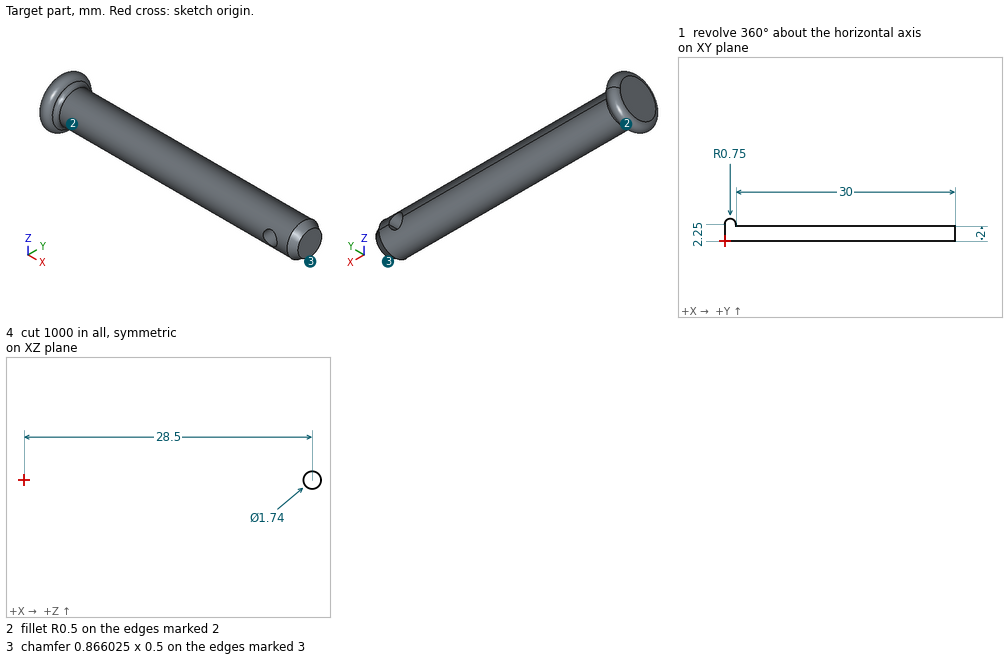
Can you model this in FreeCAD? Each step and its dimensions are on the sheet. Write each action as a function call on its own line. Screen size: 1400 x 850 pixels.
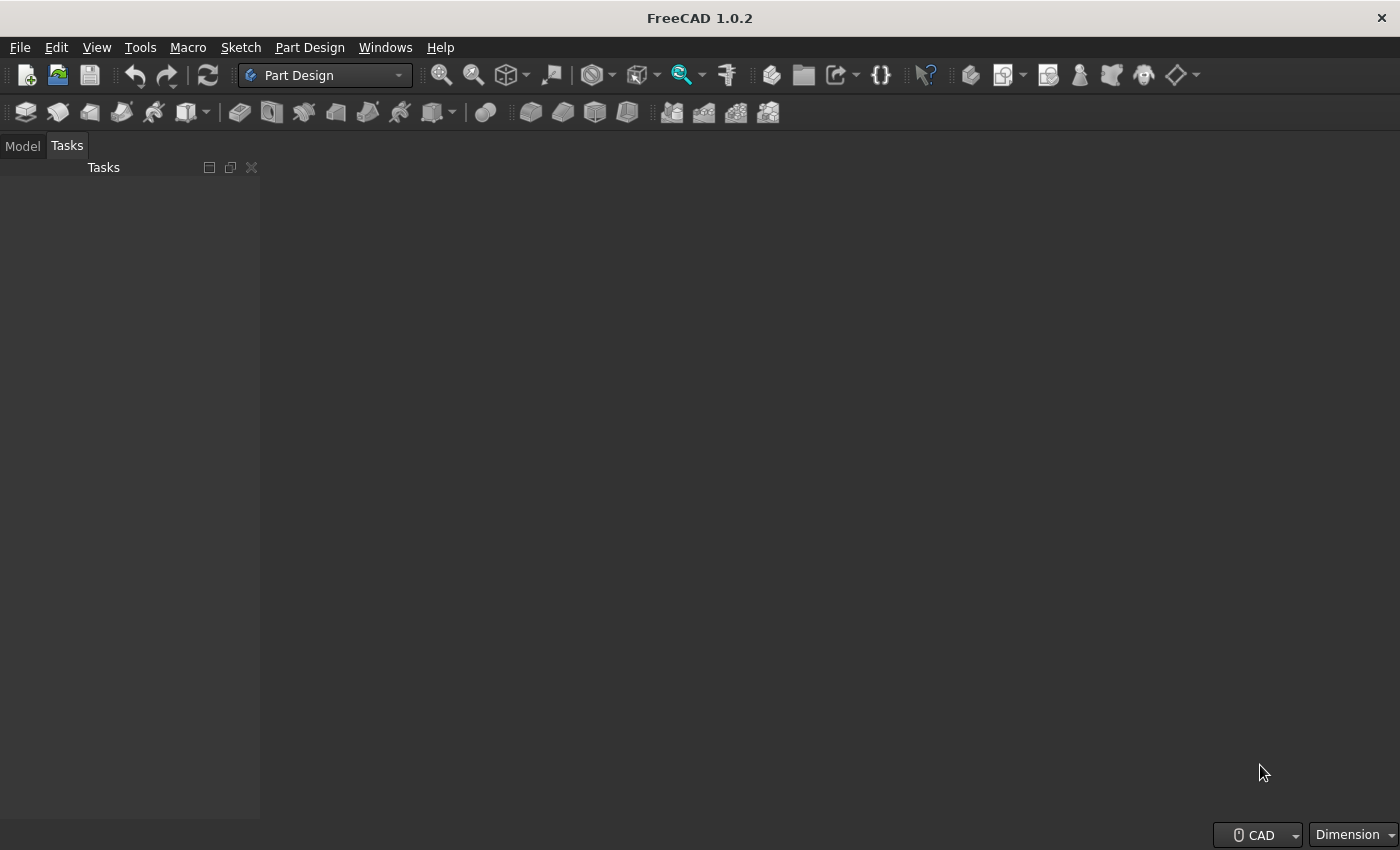
click(26, 76)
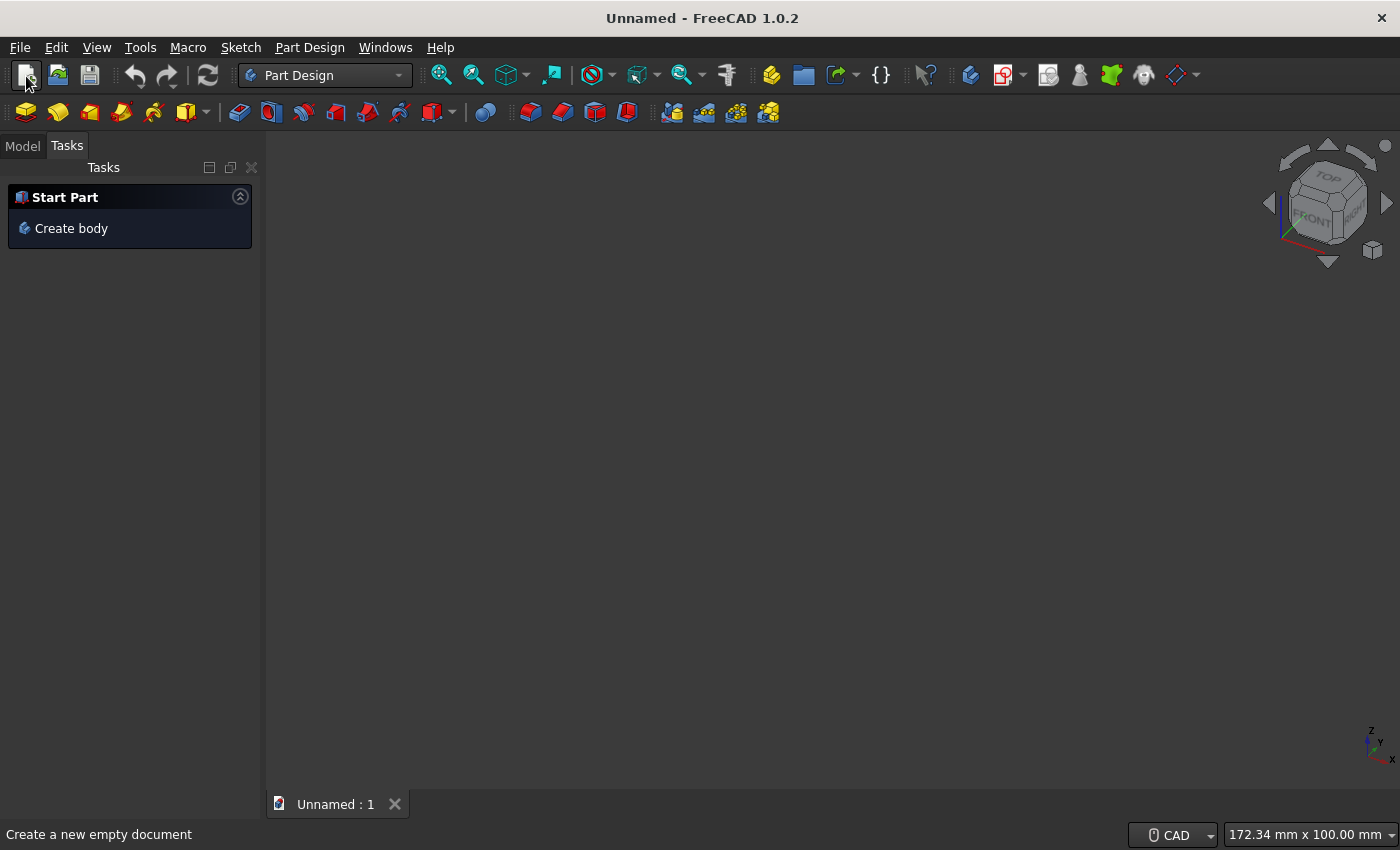
click(1004, 76)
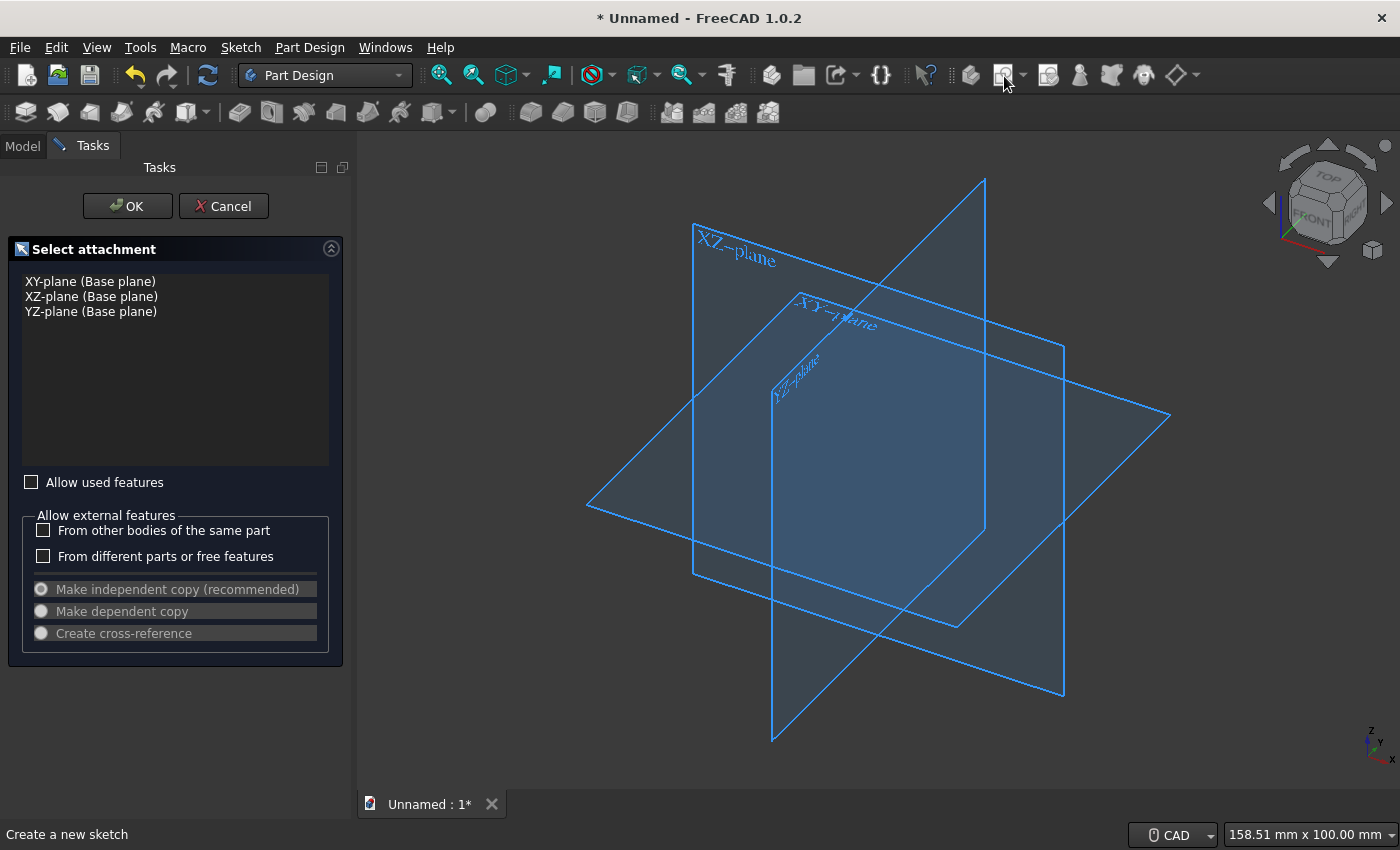
click(82, 282)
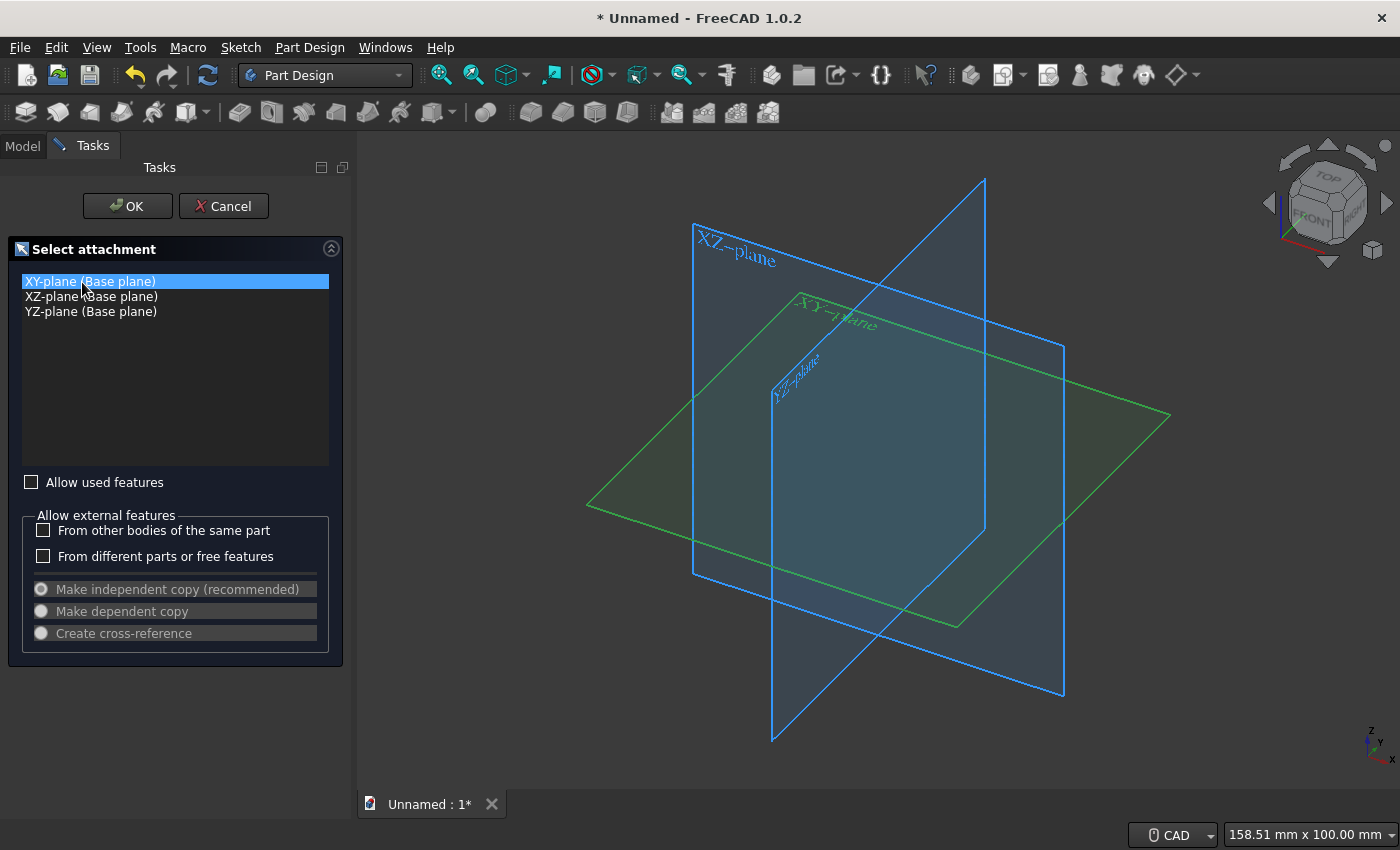
click(128, 206)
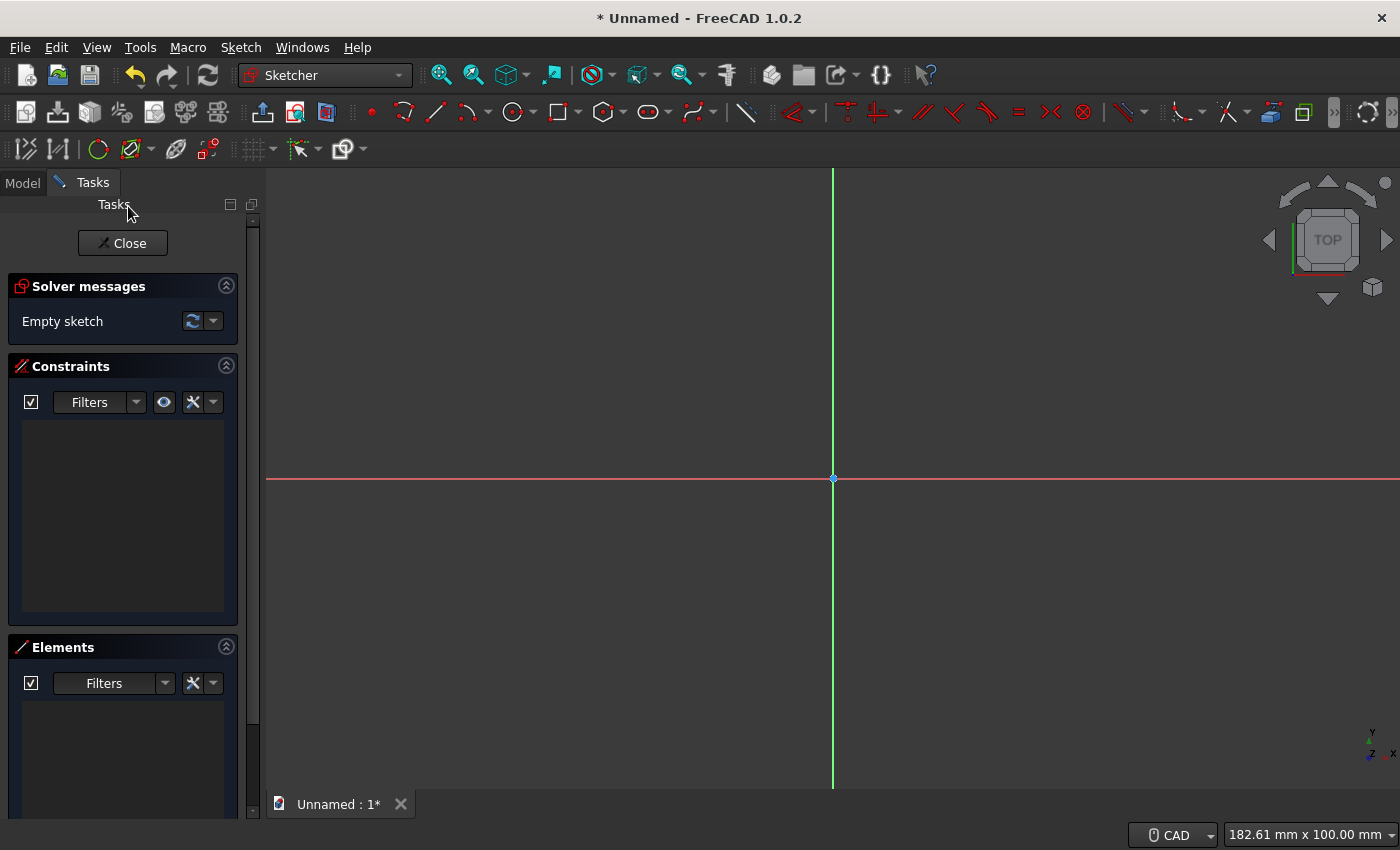
scroll(1002, 465, up, 6)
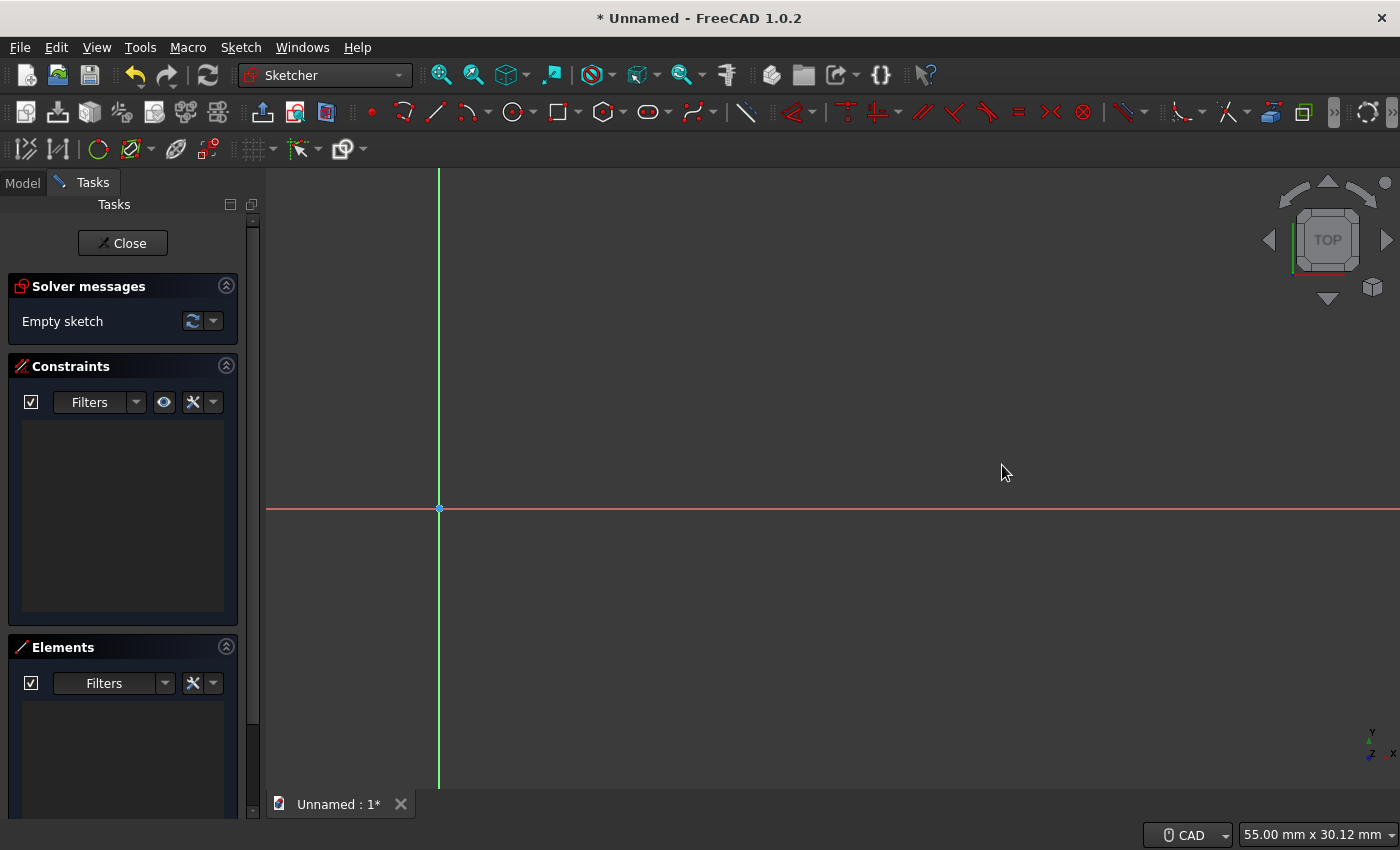
key(g)
key(m)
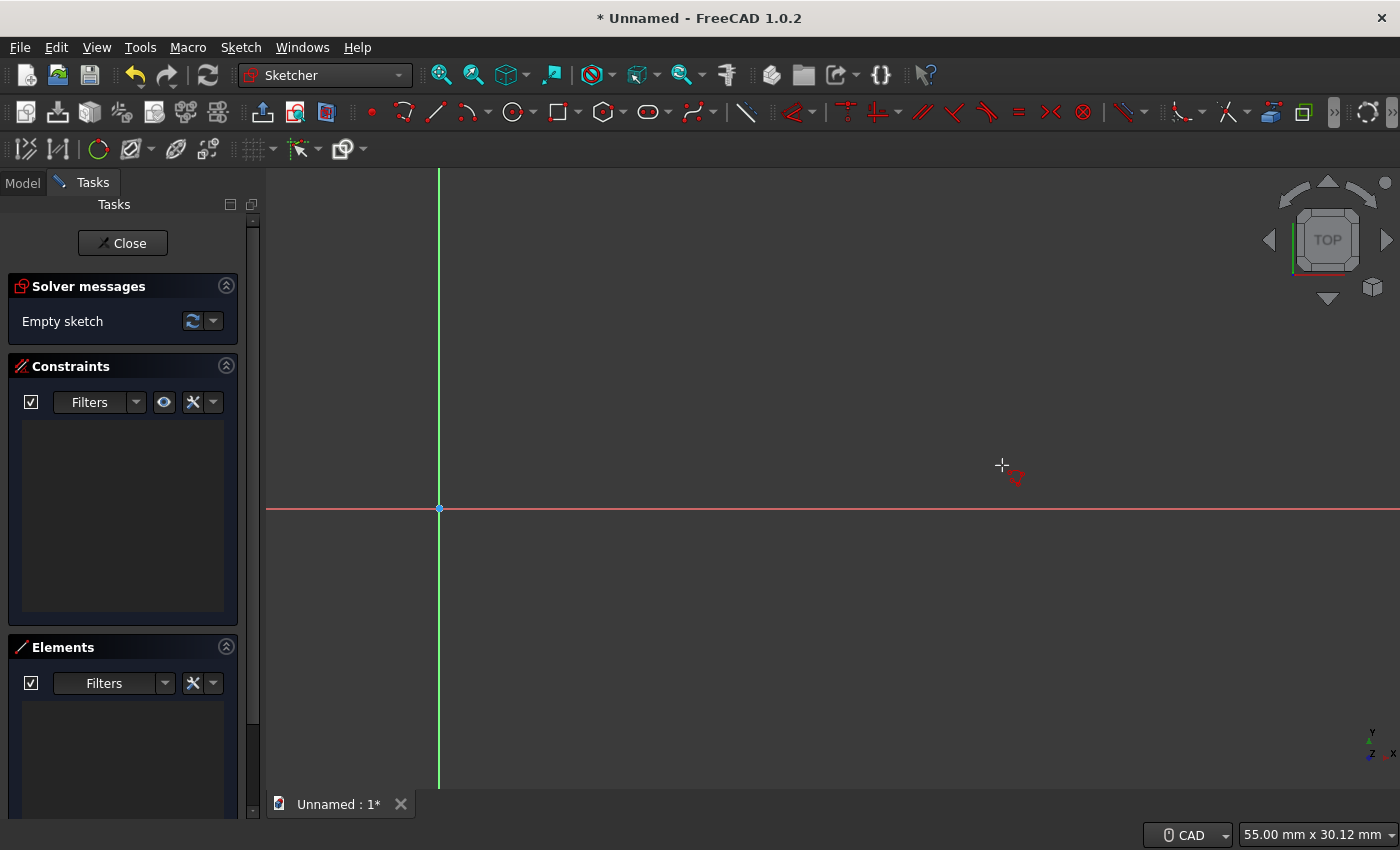
click(439, 462)
click(439, 509)
click(1089, 500)
click(1089, 467)
click(470, 467)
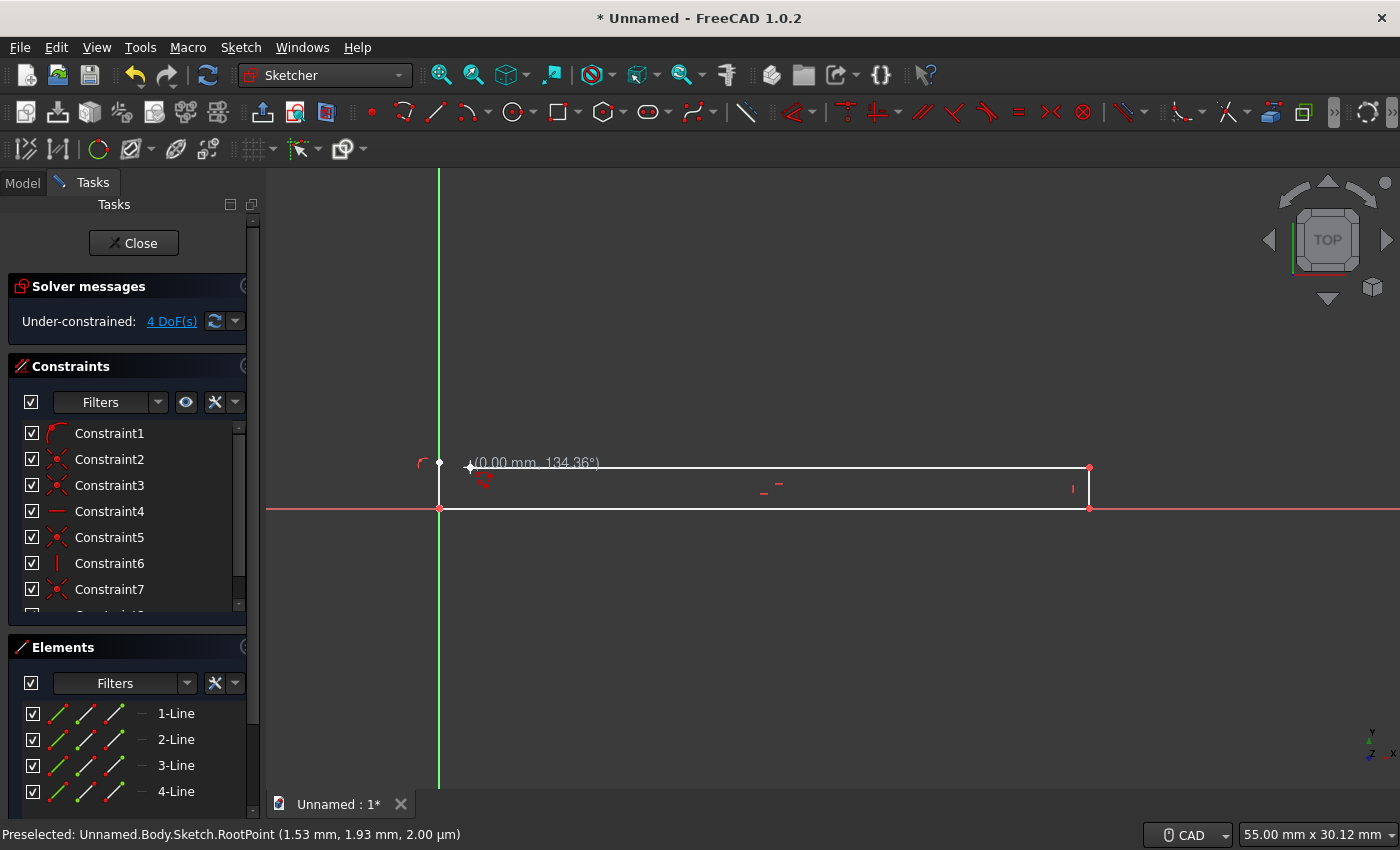
scroll(470, 462, up, 6)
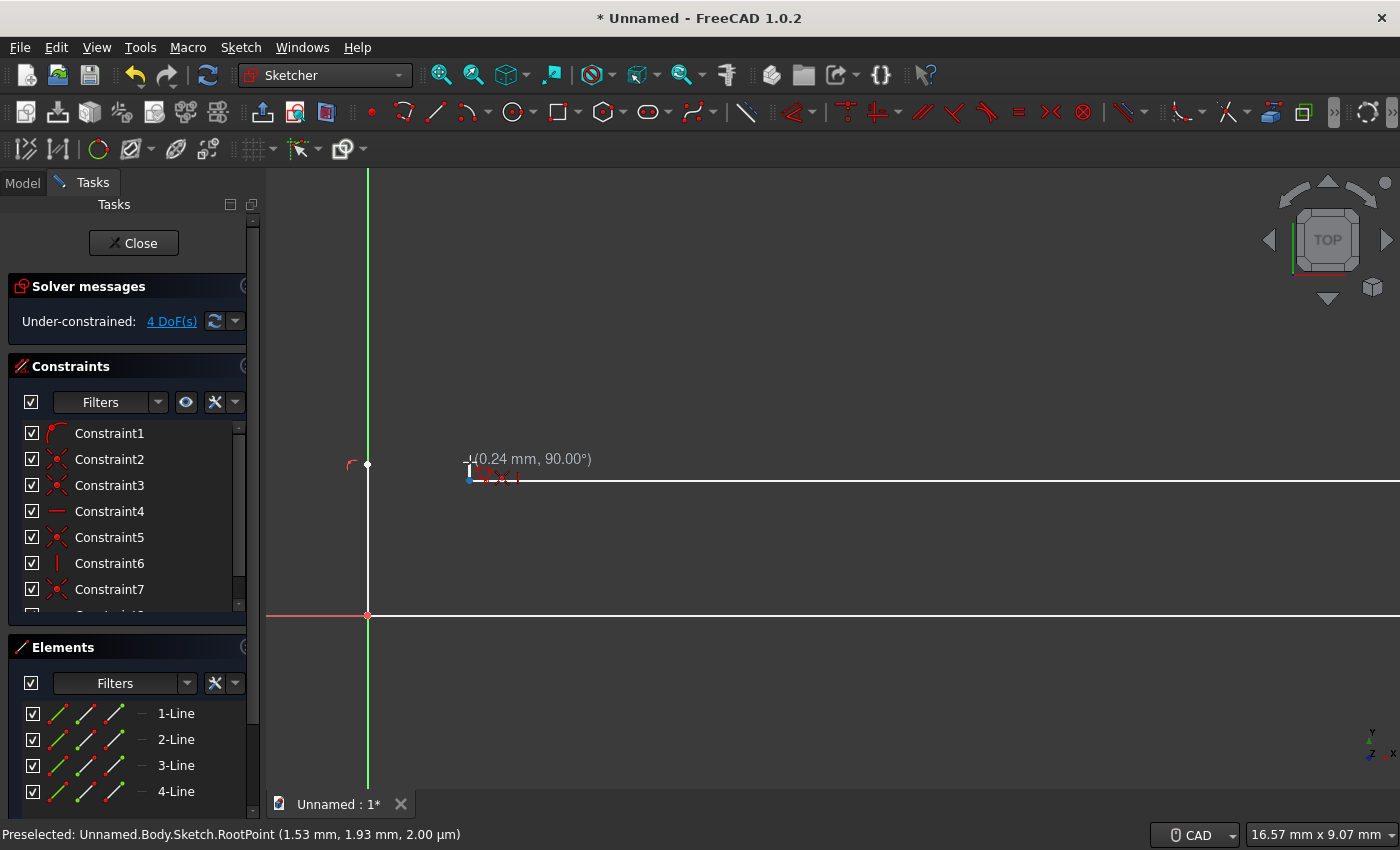
click(470, 462)
right_click(470, 462)